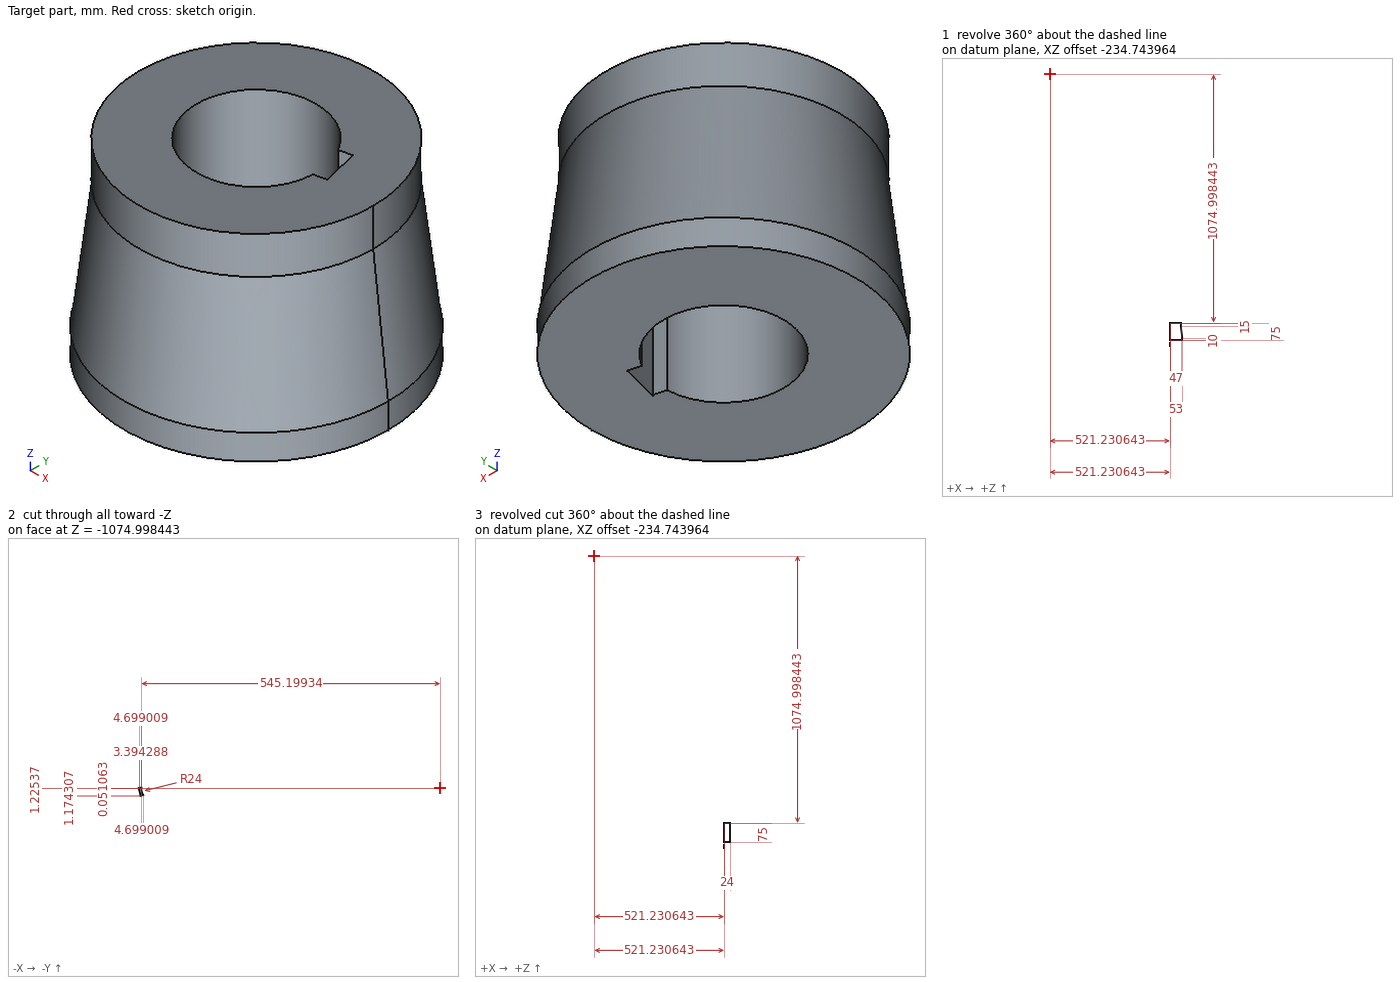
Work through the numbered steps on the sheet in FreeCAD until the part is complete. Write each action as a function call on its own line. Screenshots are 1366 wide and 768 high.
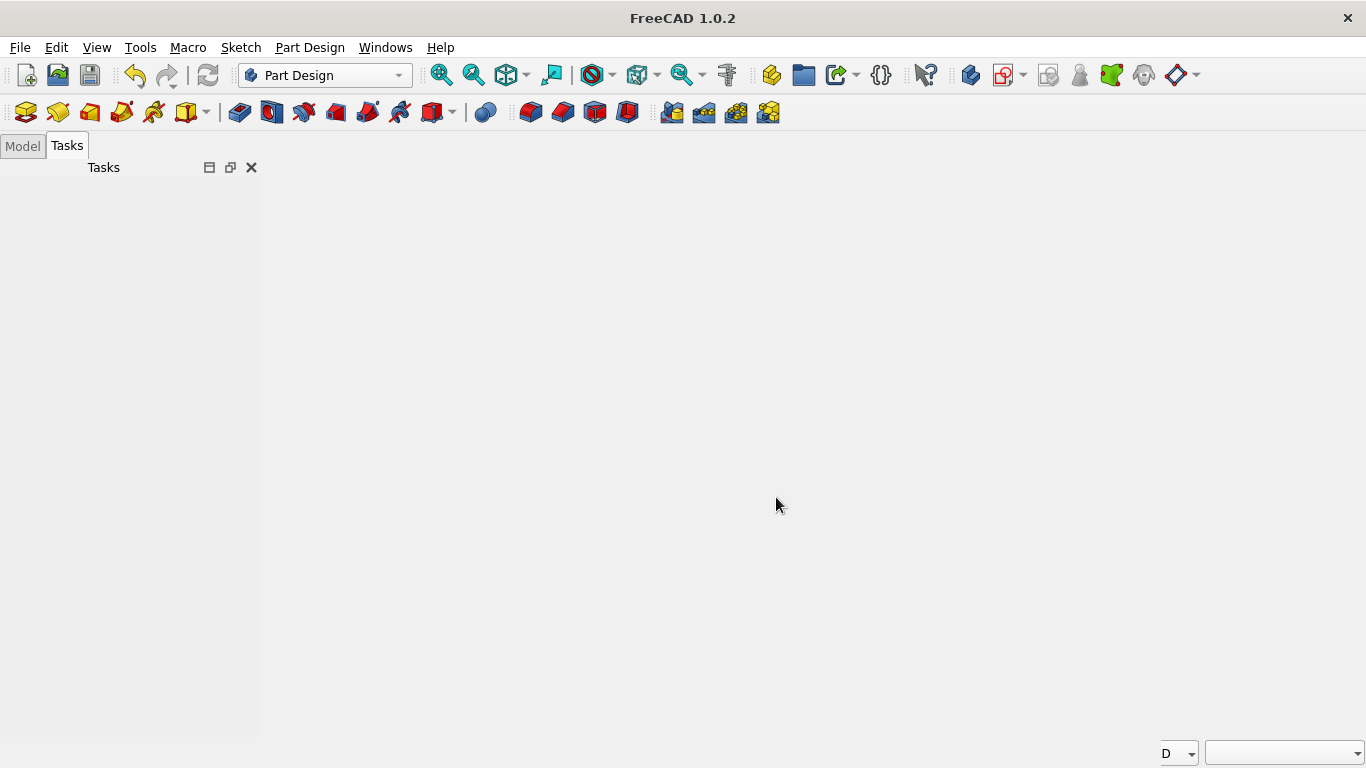
click(26, 76)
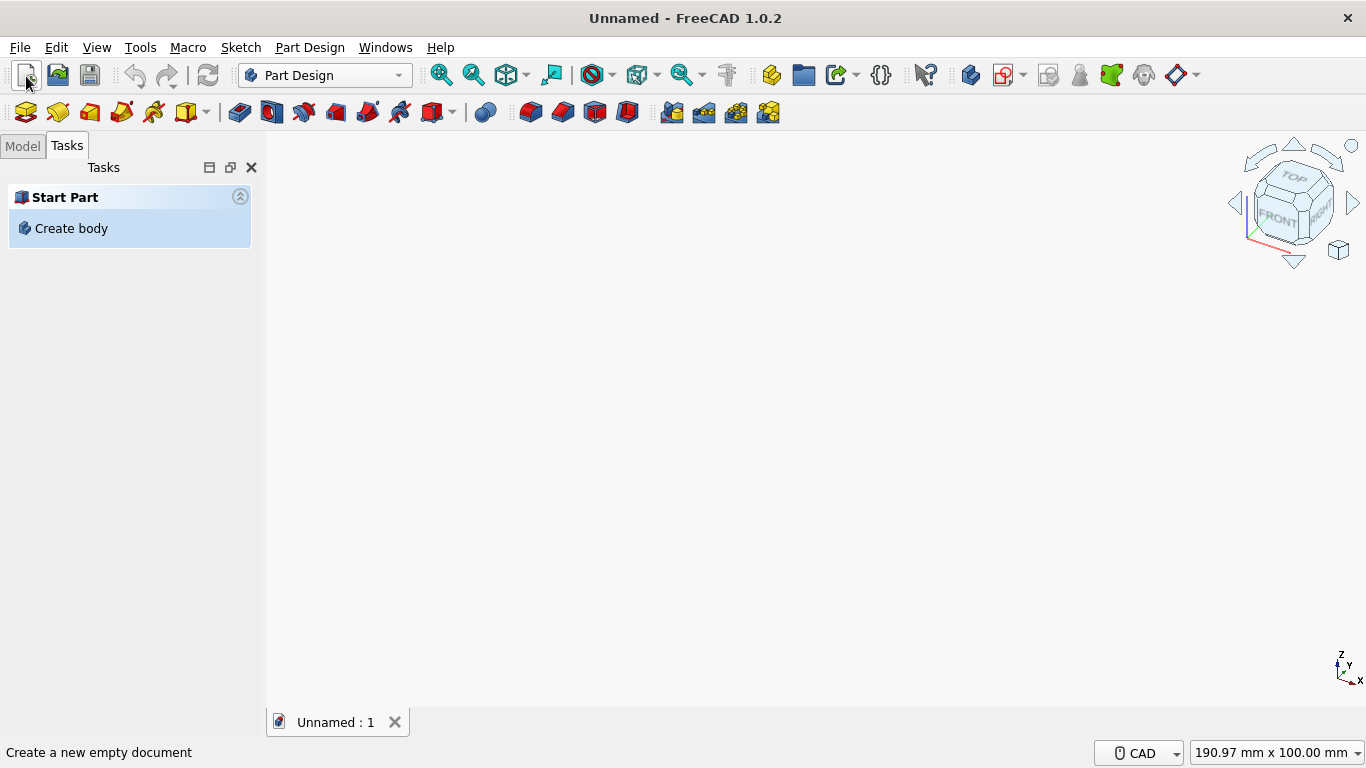
click(972, 76)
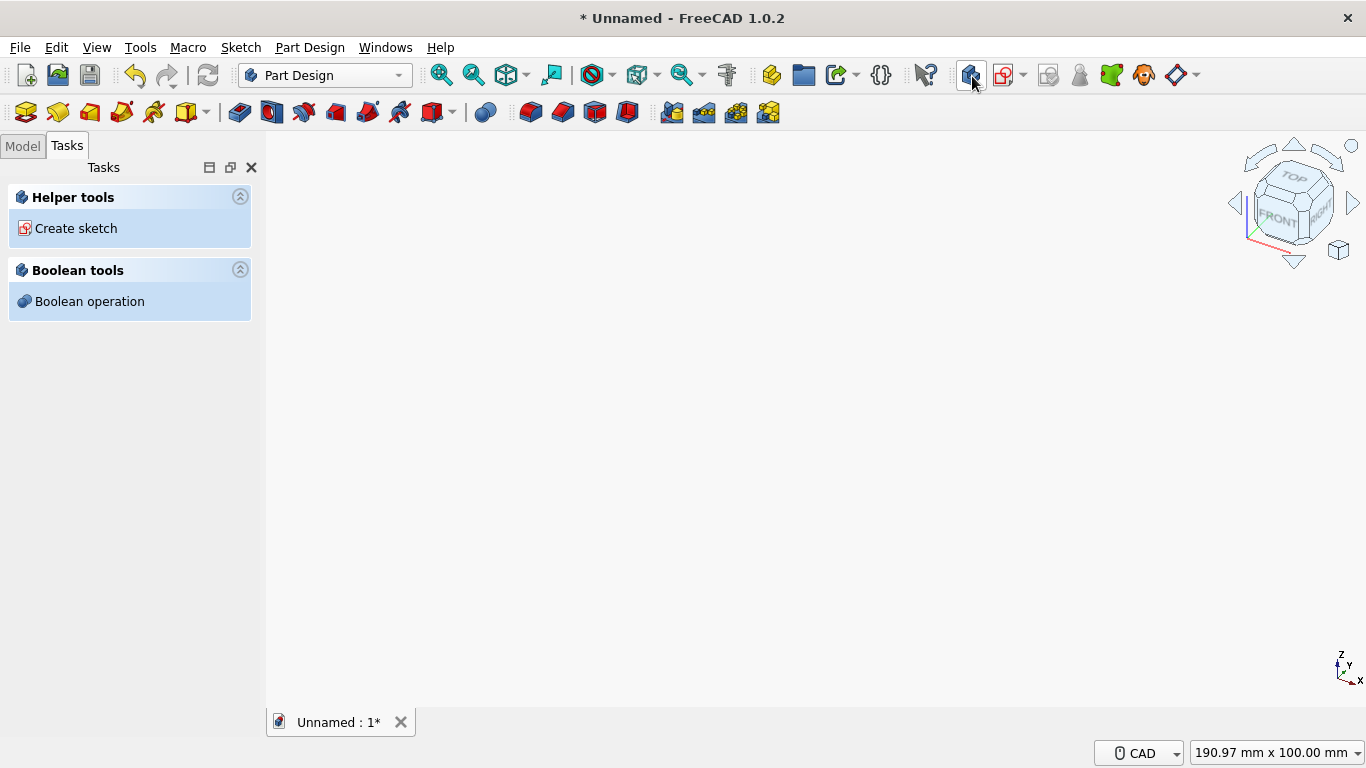
click(23, 145)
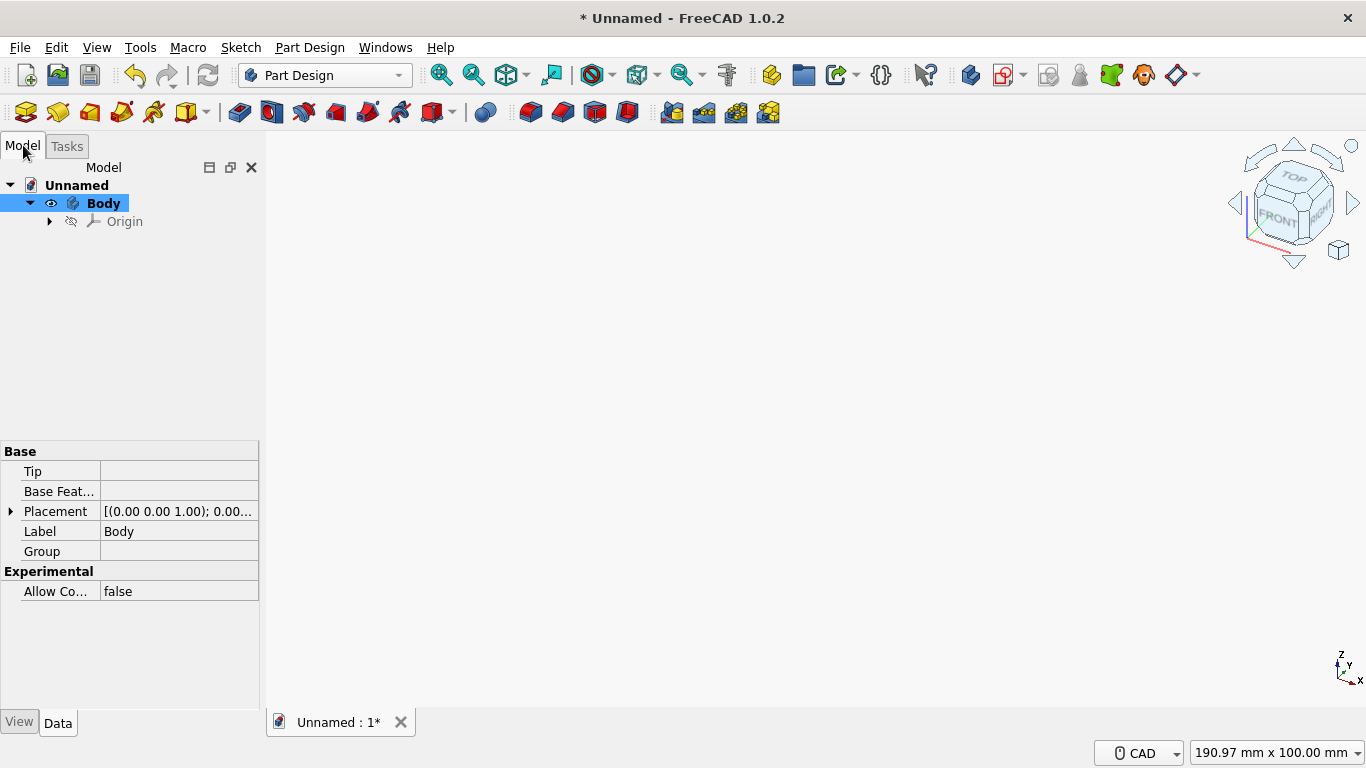
click(50, 221)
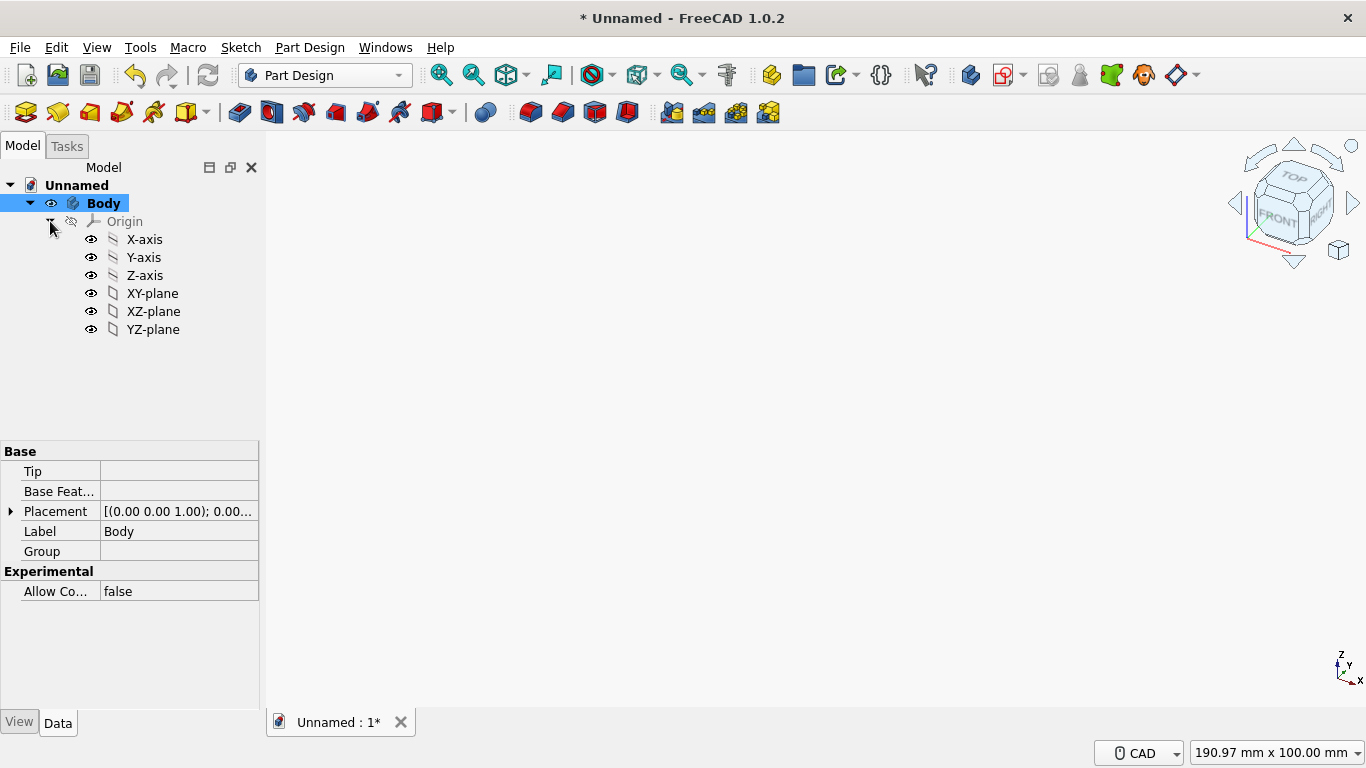
click(136, 311)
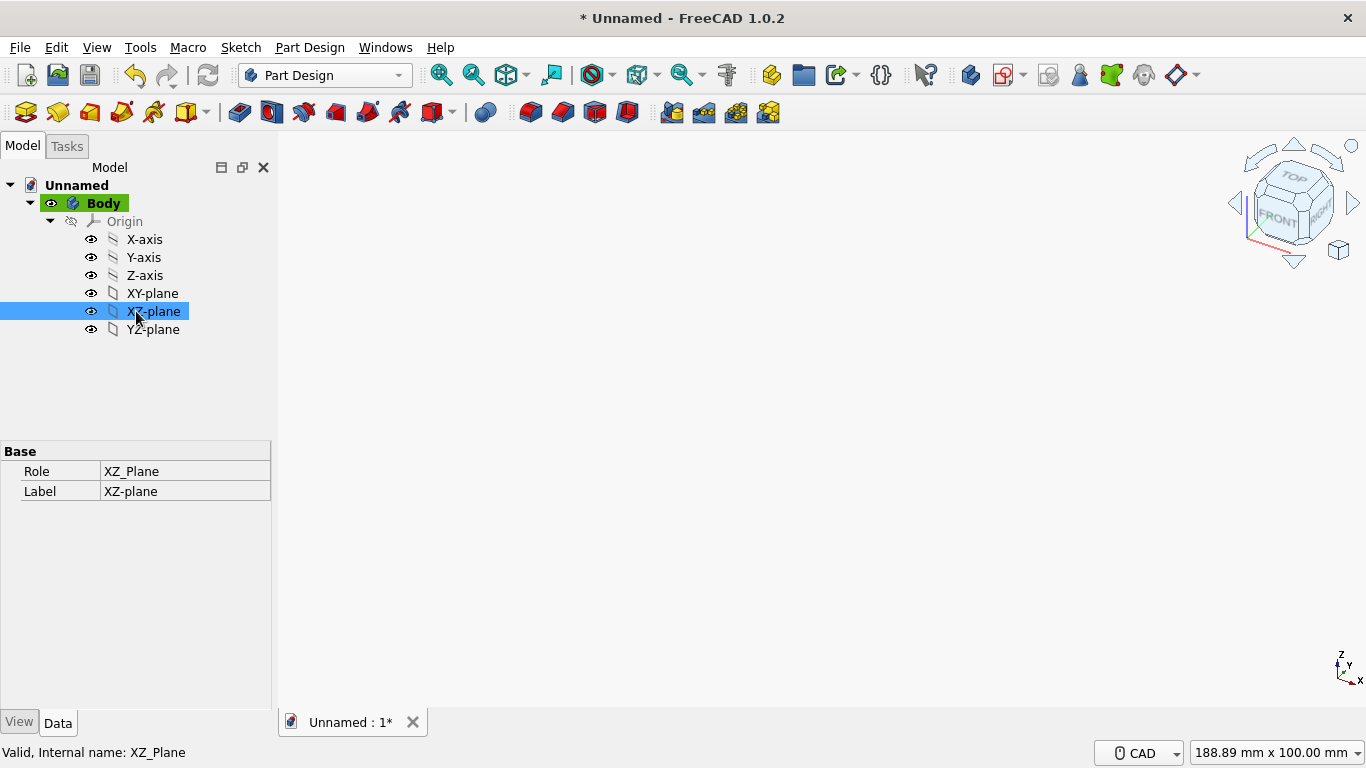
click(1176, 76)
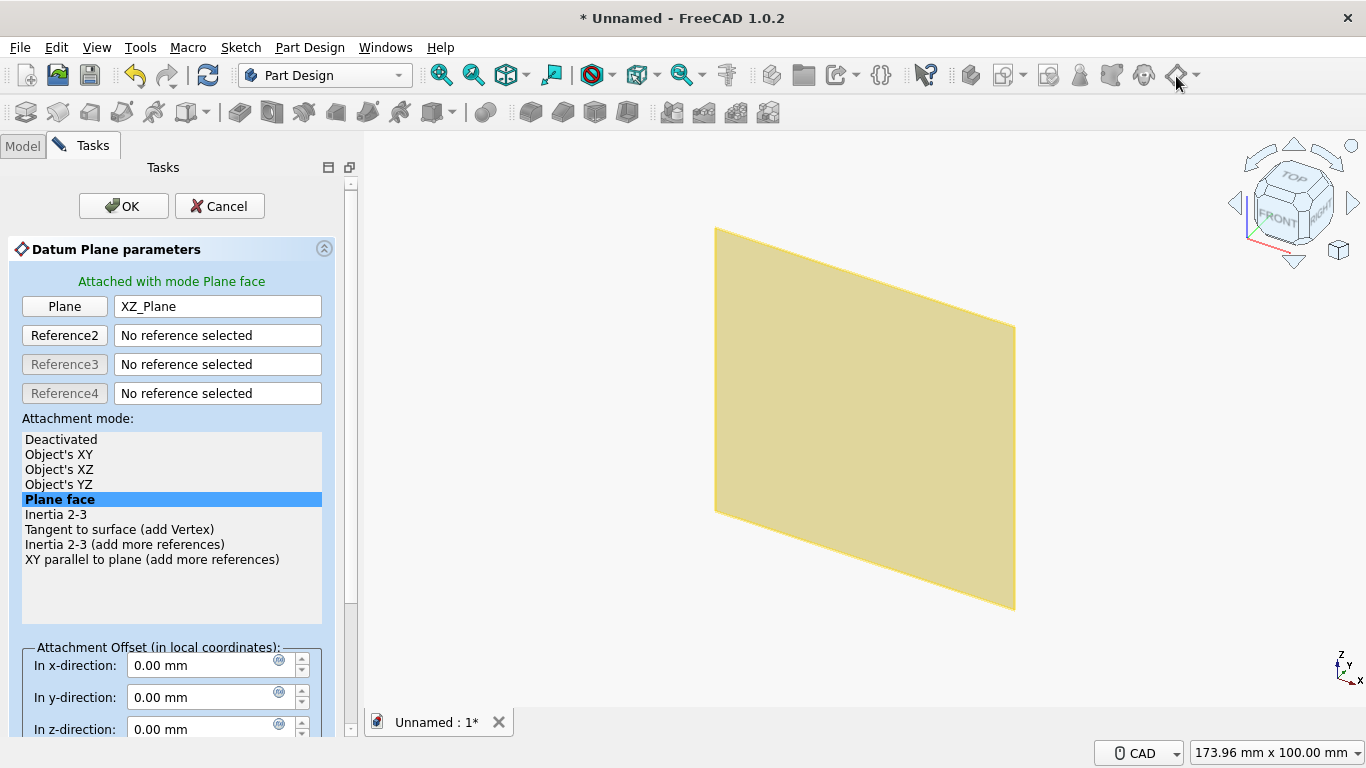
scroll(351, 456, down, 2)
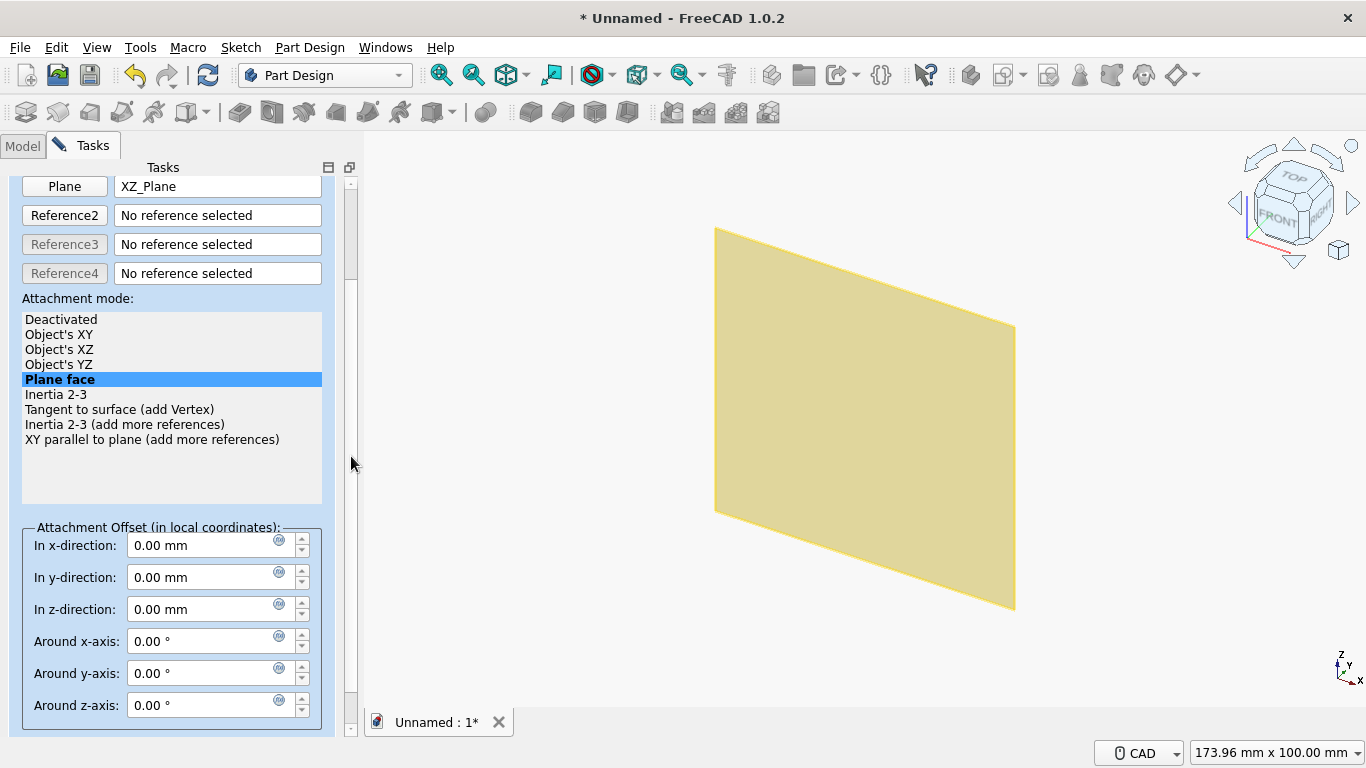
triple_click(210, 609)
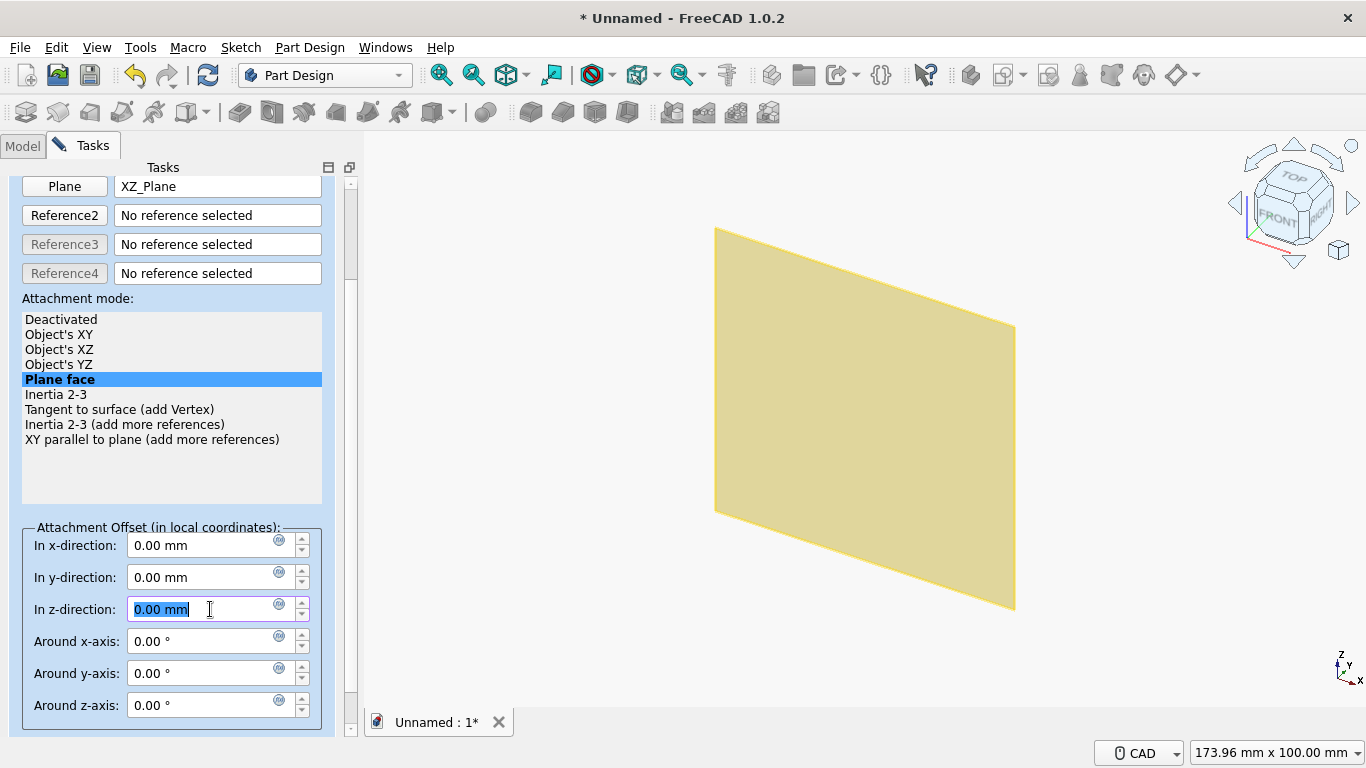
text(-234.743964)
key(Tab)